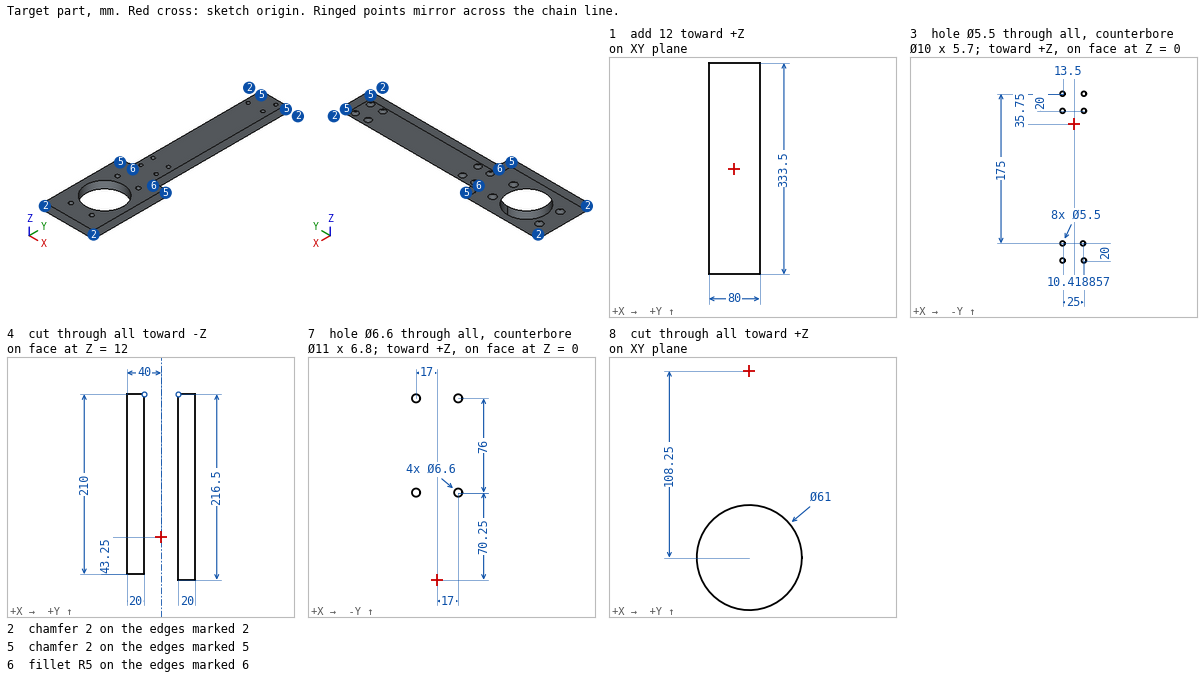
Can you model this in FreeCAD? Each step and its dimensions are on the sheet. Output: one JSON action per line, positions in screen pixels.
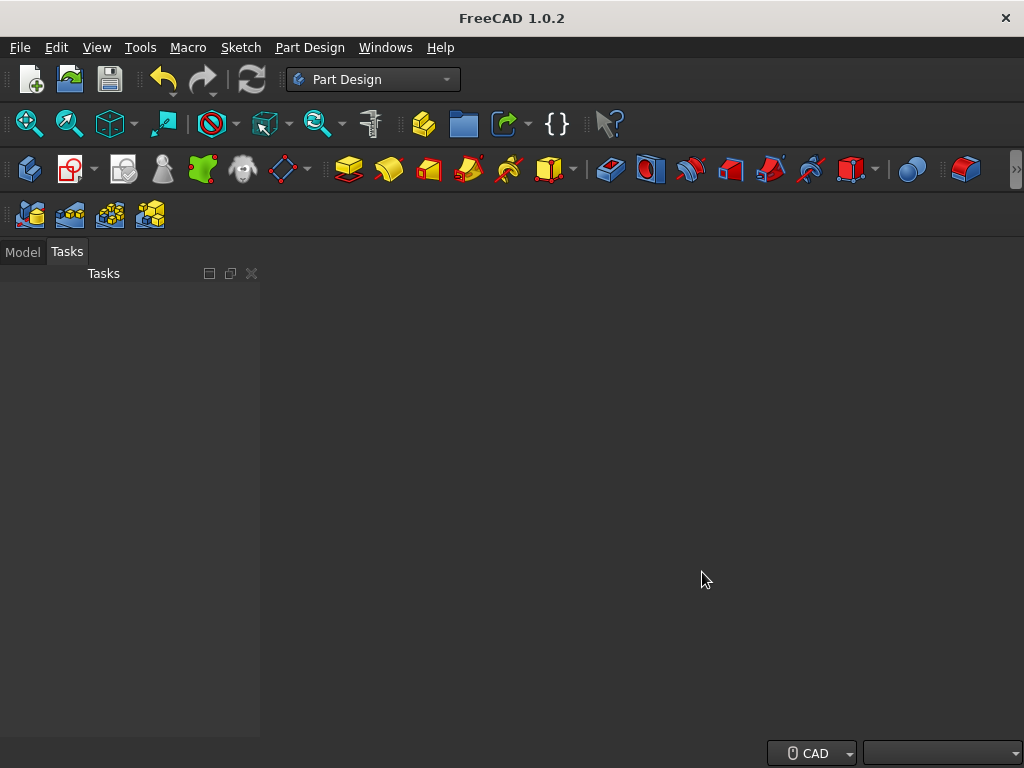
{"action": "key", "text": "ctrl+n"}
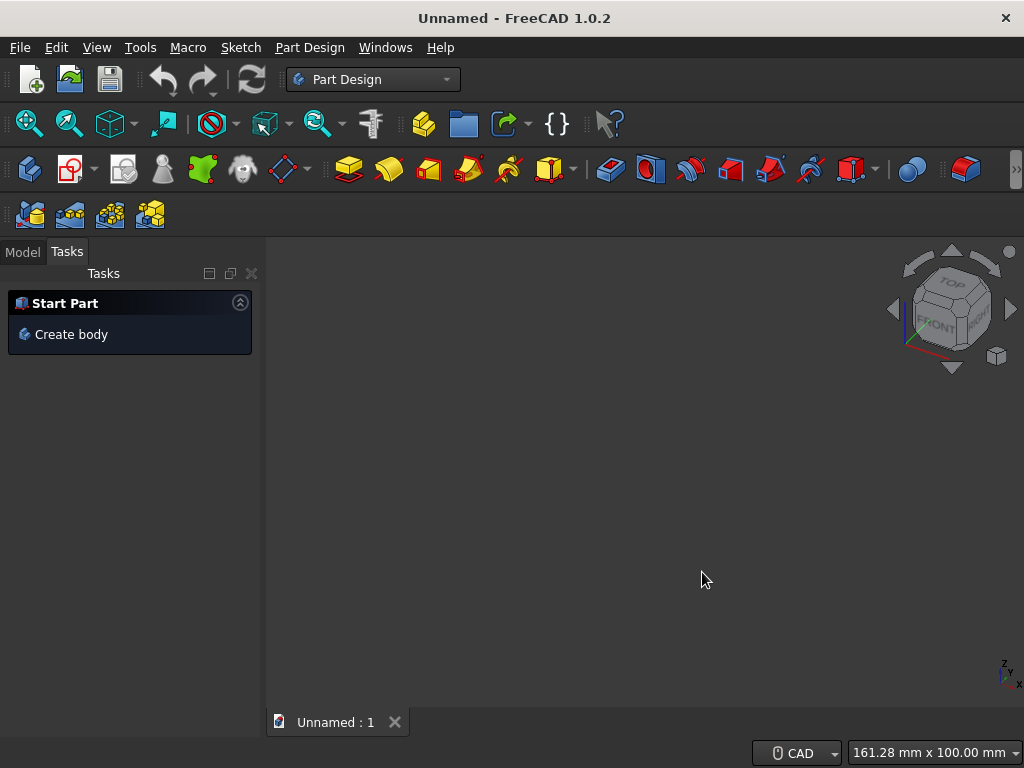
{"action": "left_click", "coordinate": [70, 170]}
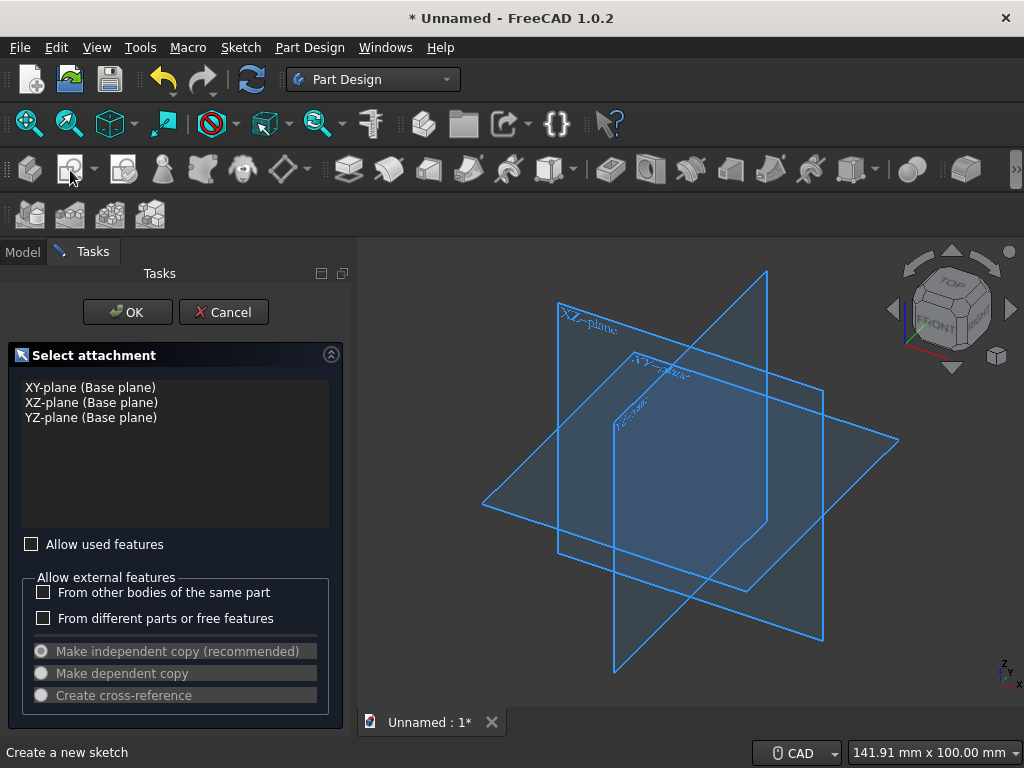
{"action": "left_click", "coordinate": [82, 388]}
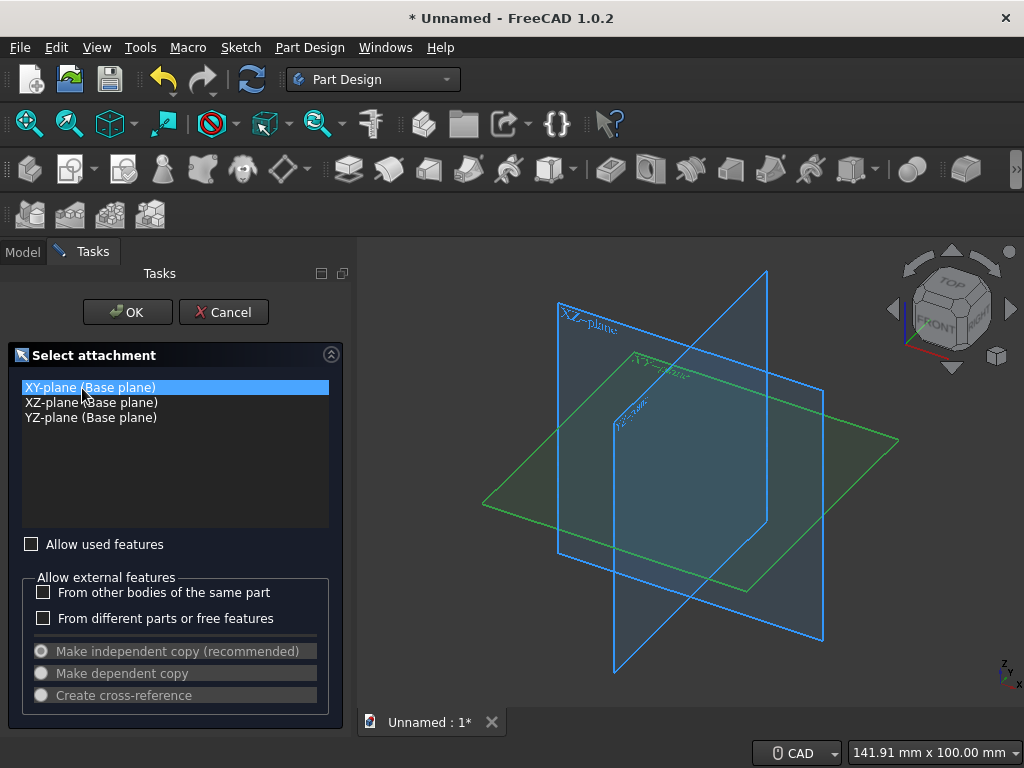
{"action": "left_click", "coordinate": [128, 312]}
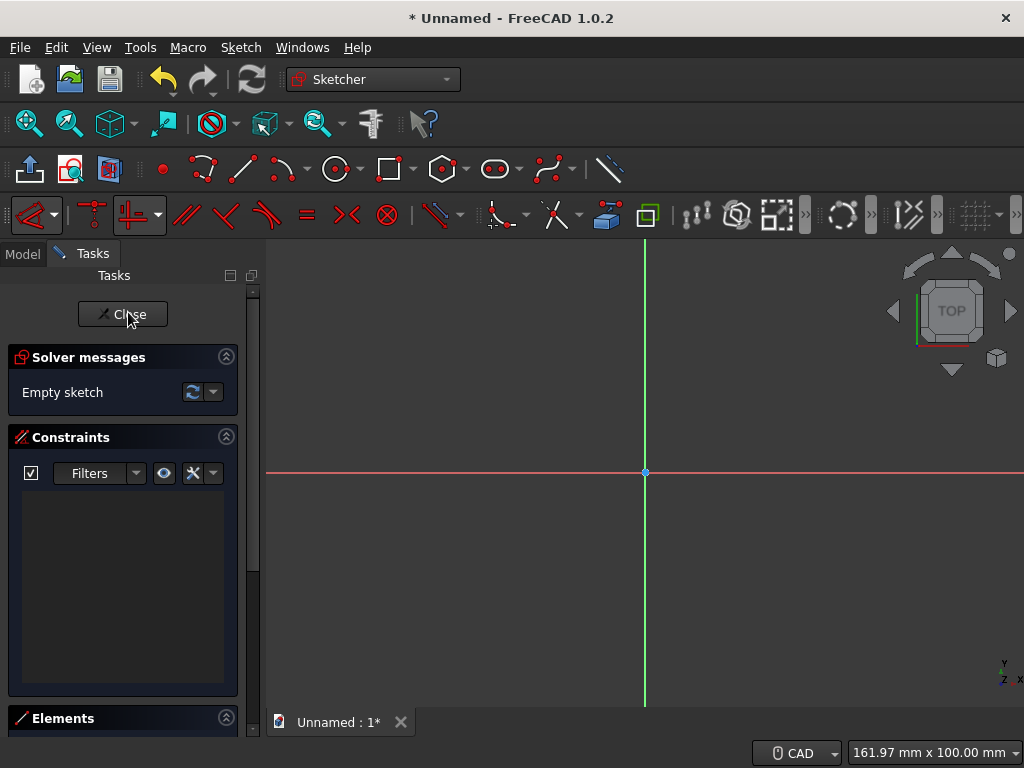
{"action": "scroll", "coordinate": [559, 473], "scroll_direction": "down", "scroll_amount": 8}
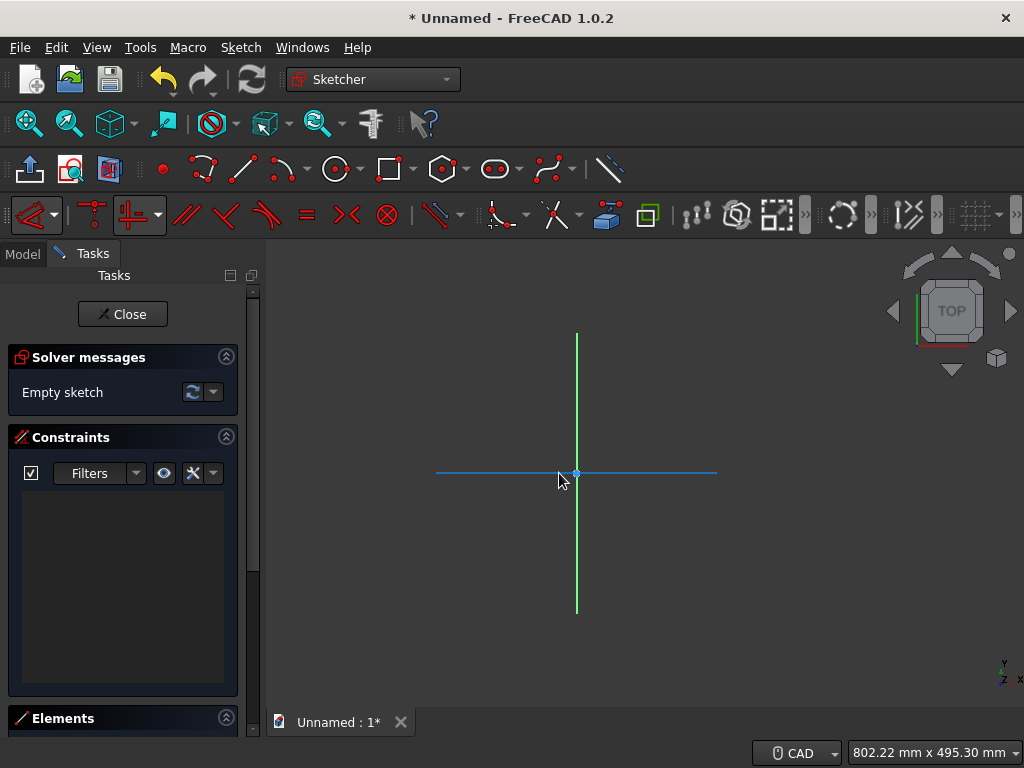
{"action": "key", "text": "g v"}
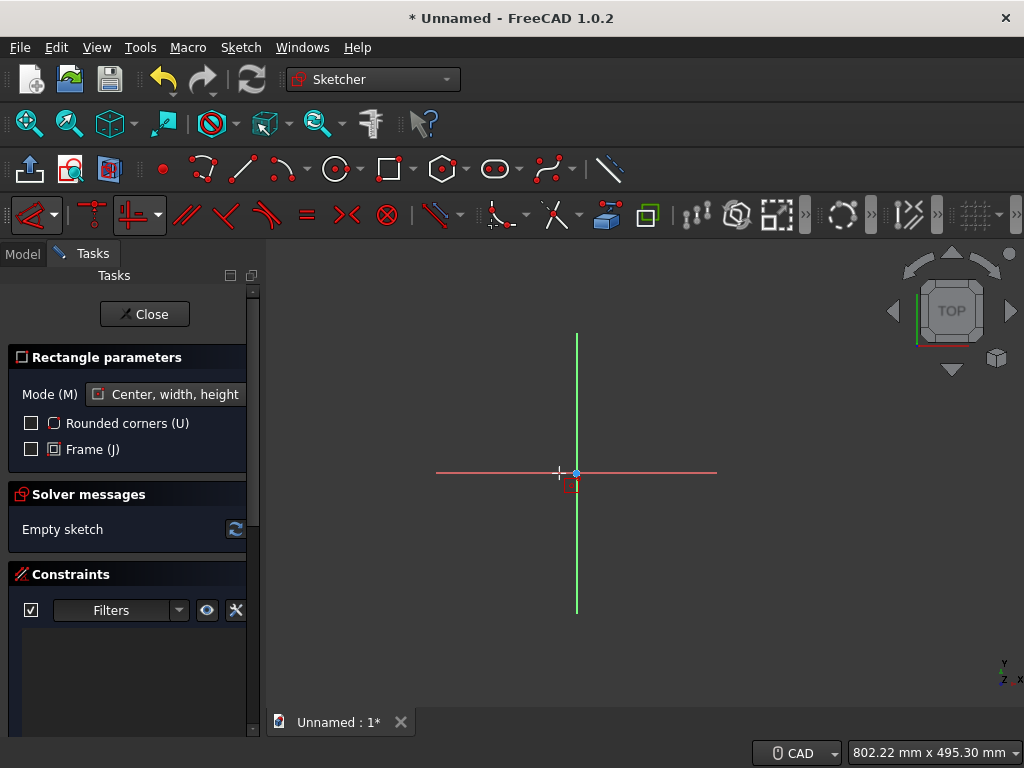
{"action": "left_click", "coordinate": [577, 473]}
{"action": "left_click", "coordinate": [614, 316]}
{"action": "key", "text": "Escape"}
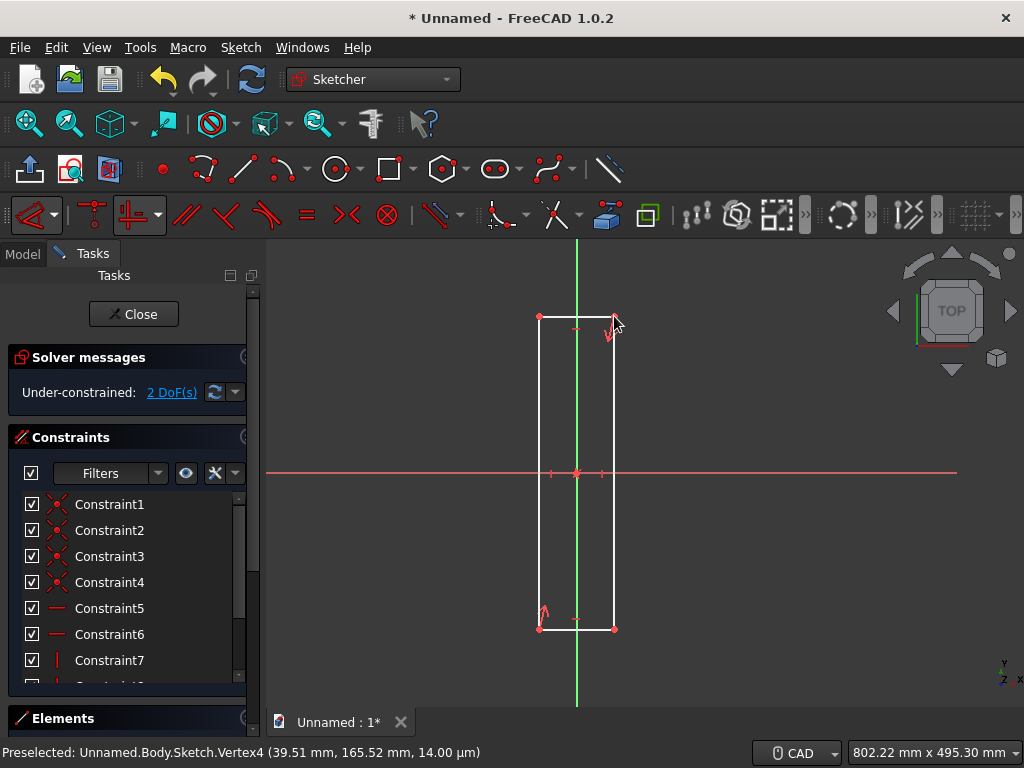
{"action": "key", "text": "d"}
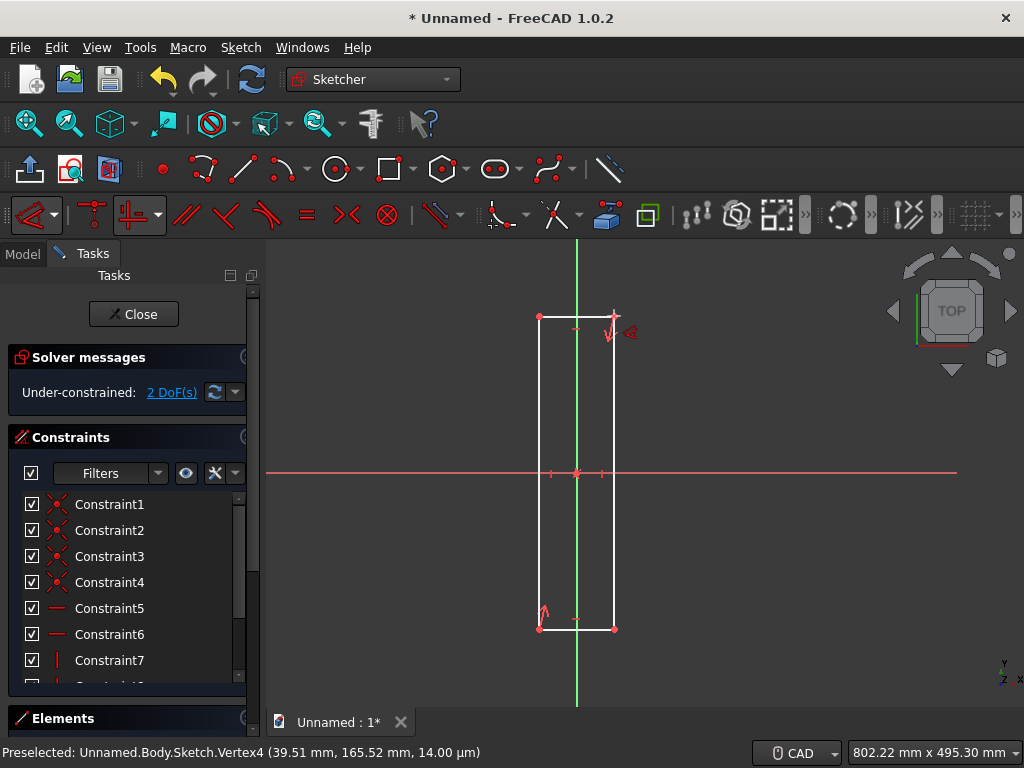
{"action": "left_click", "coordinate": [562, 630]}
{"action": "left_click", "coordinate": [560, 664]}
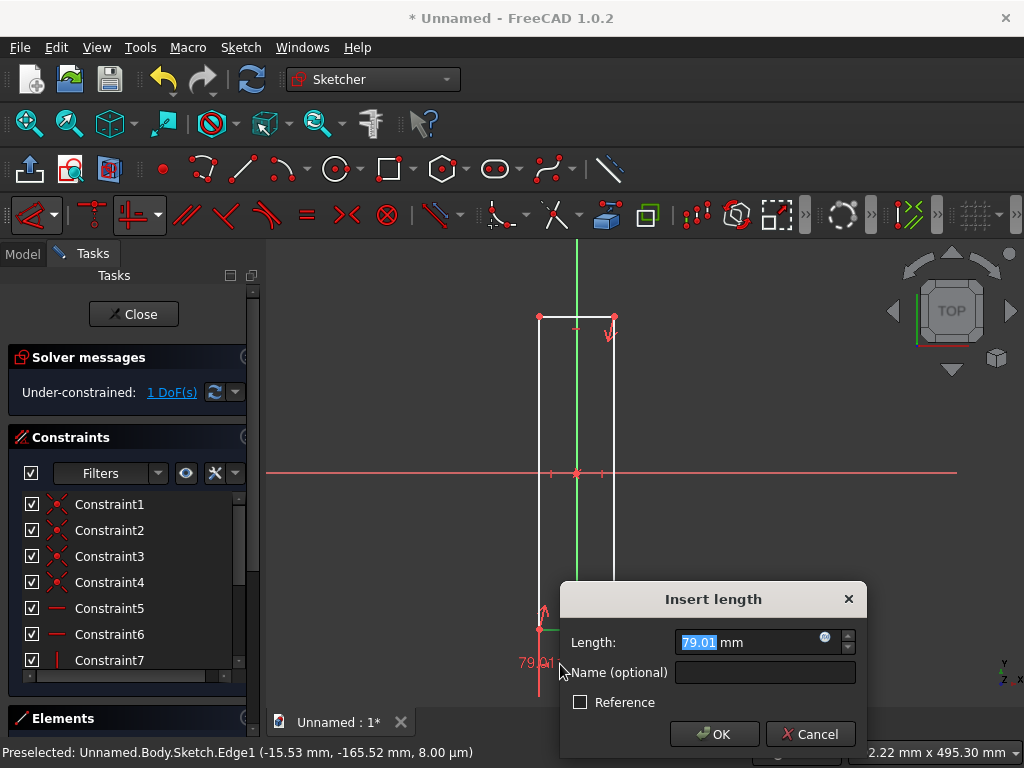
{"action": "type", "text": "80"}
{"action": "key", "text": "Return"}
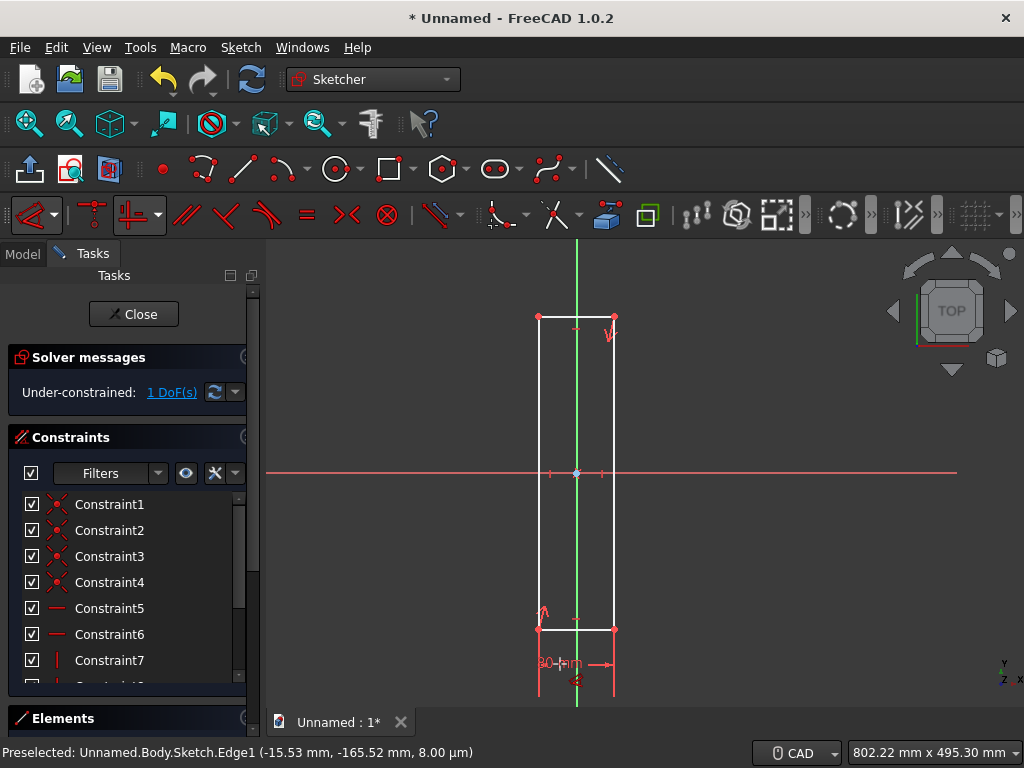
{"action": "left_click", "coordinate": [614, 536]}
{"action": "left_click", "coordinate": [648, 401]}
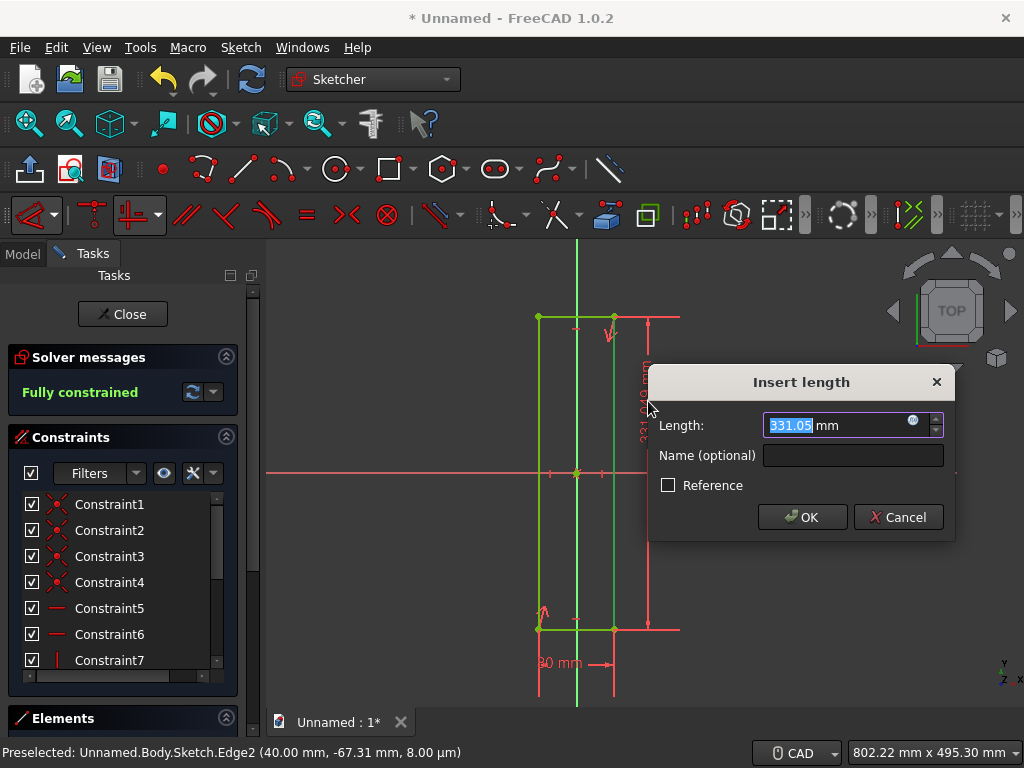
{"action": "type", "text": "333.5"}
{"action": "key", "text": "Return"}
{"action": "key", "text": "Escape"}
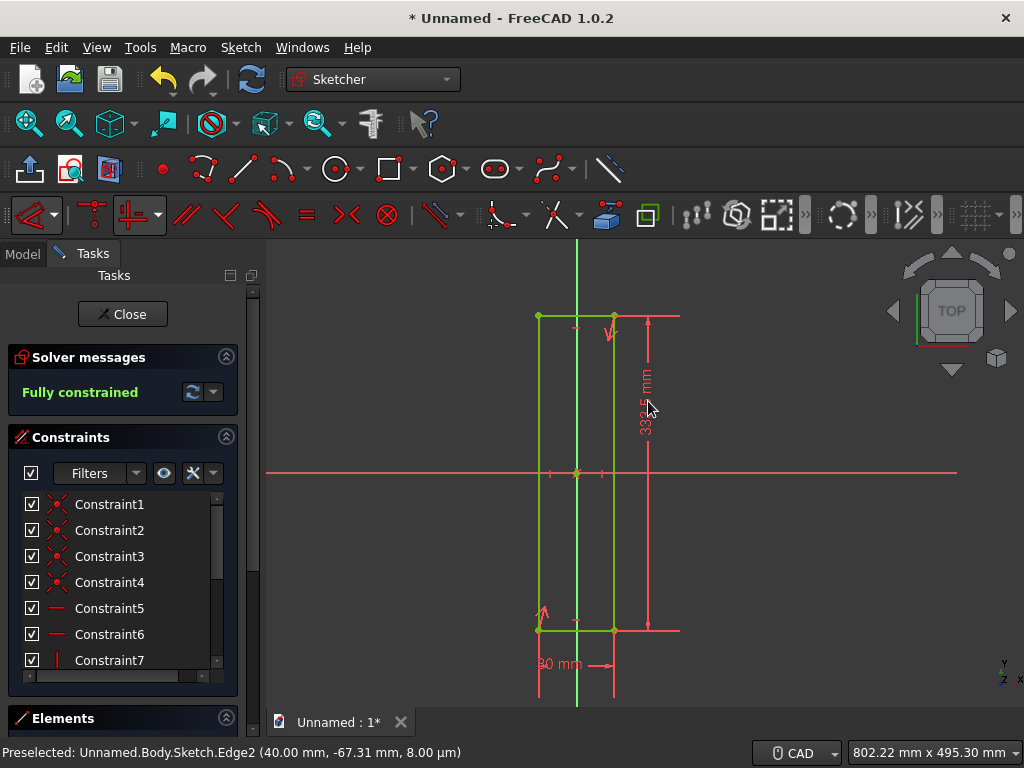
{"action": "left_click", "coordinate": [123, 314]}